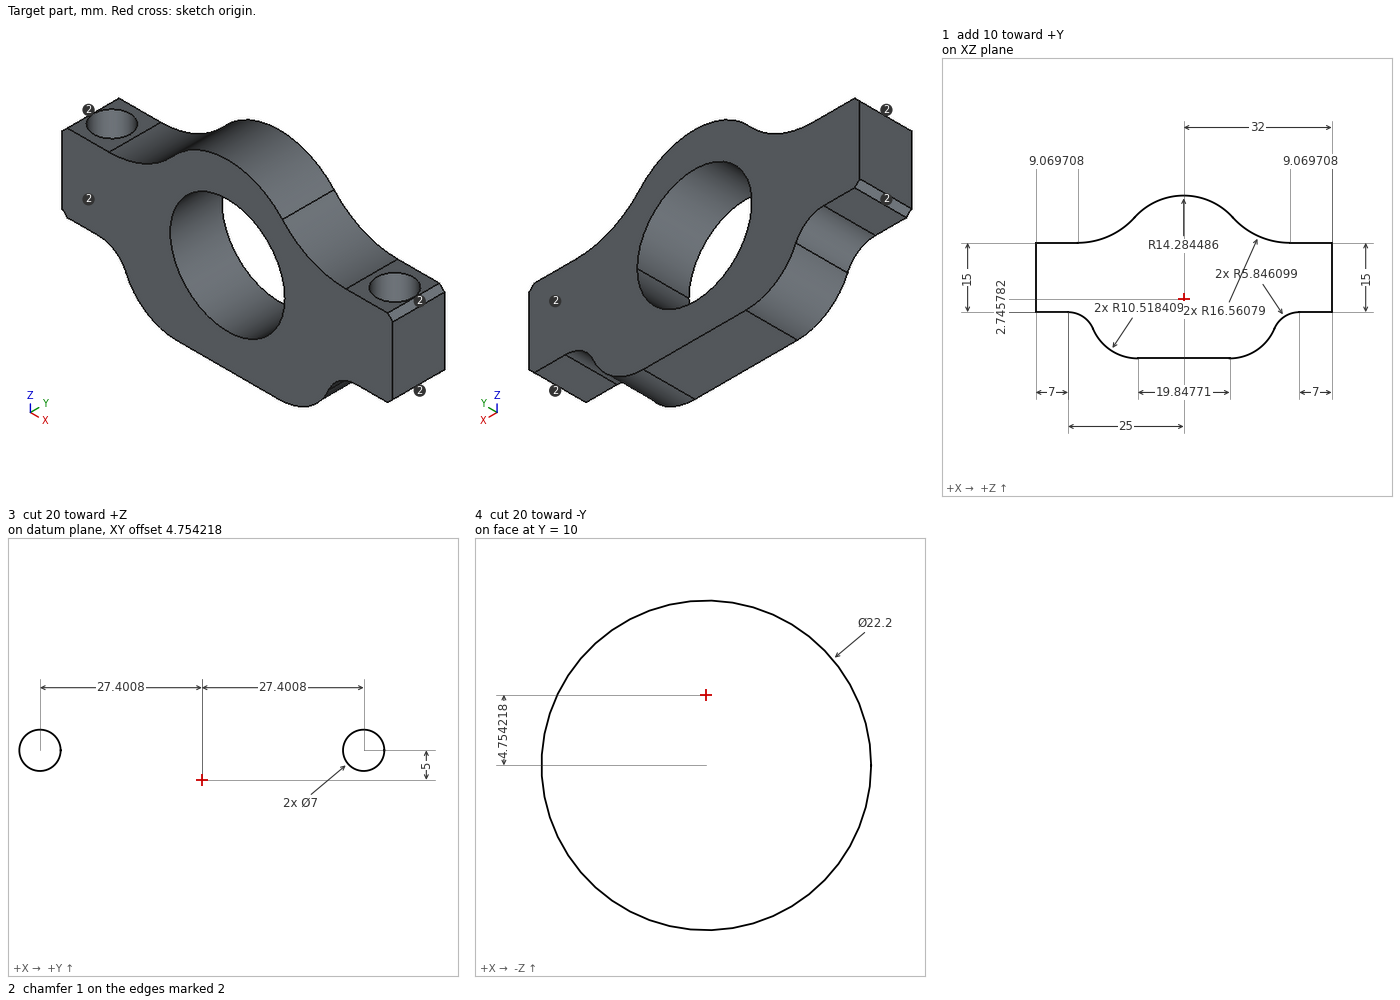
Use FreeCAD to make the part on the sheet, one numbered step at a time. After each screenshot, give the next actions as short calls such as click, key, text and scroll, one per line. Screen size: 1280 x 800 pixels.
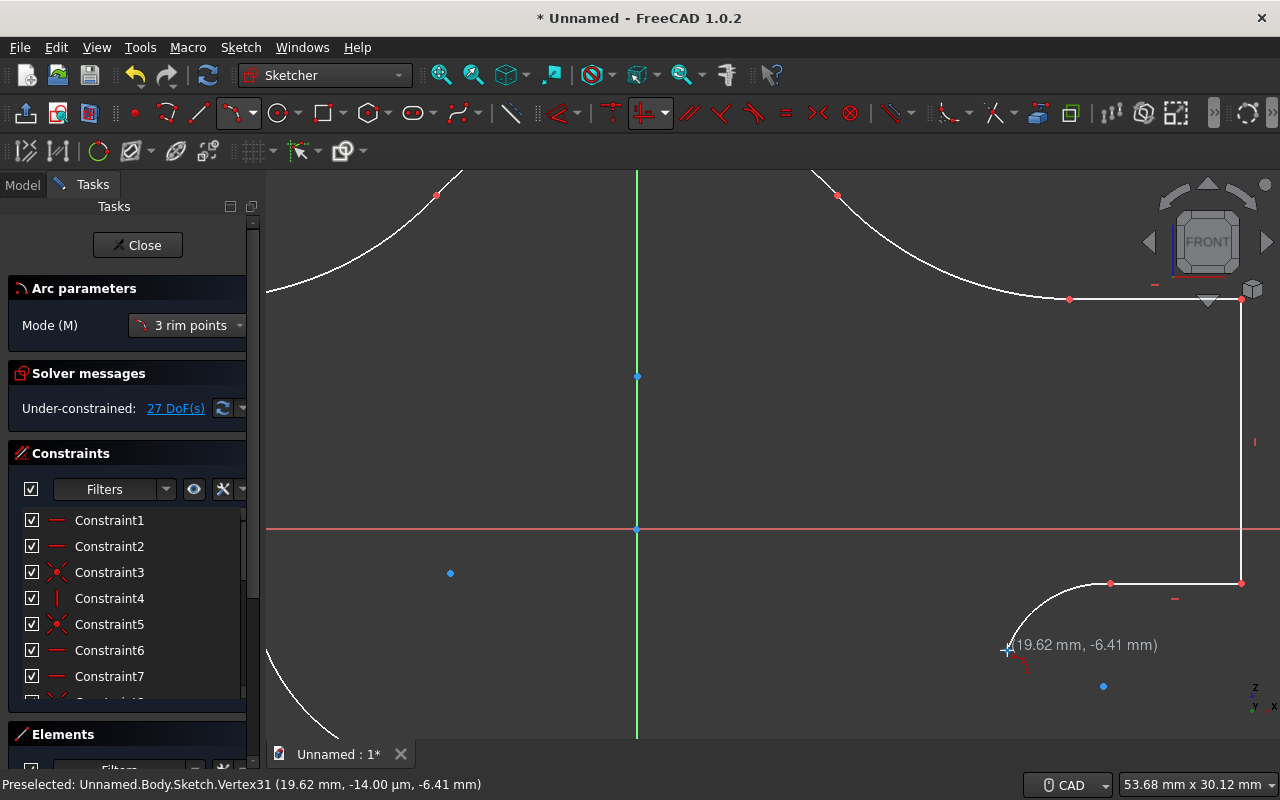
scroll(760, 468, down, 4)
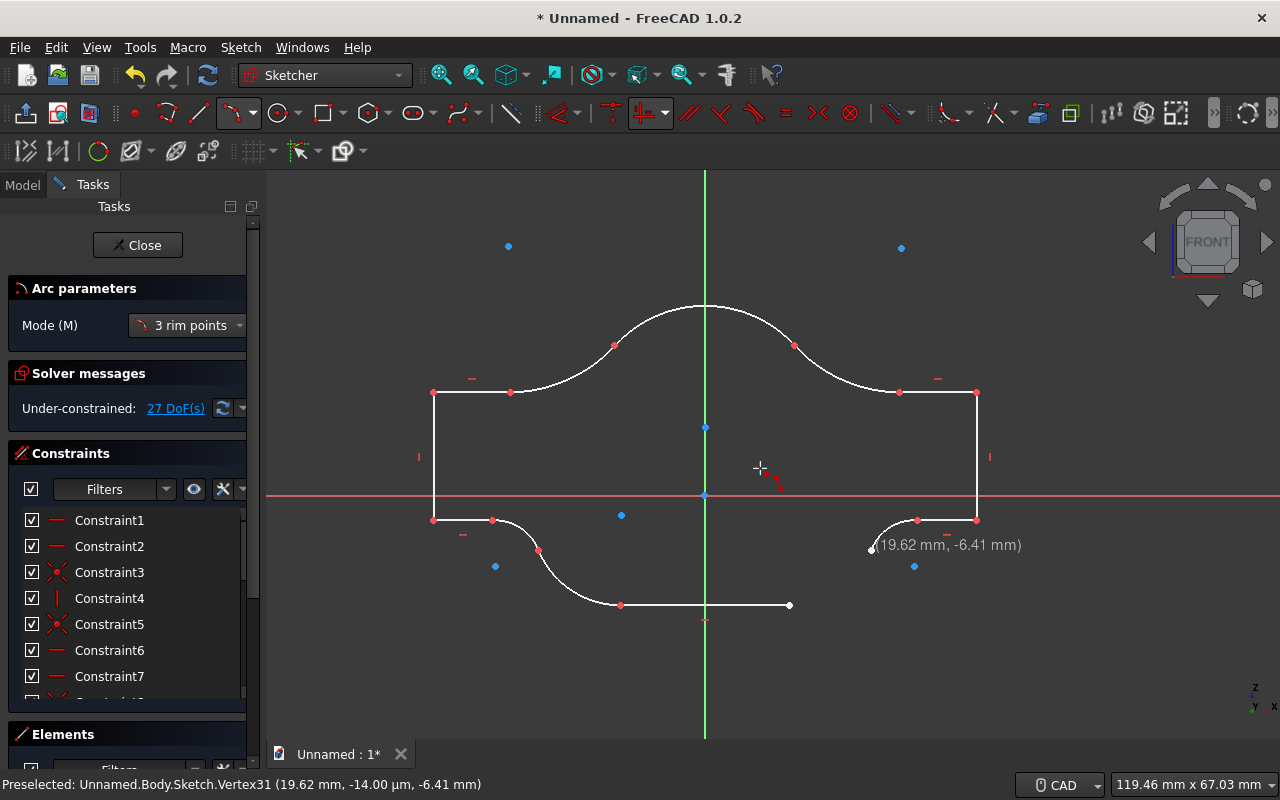
click(790, 605)
click(838, 589)
key(Escape)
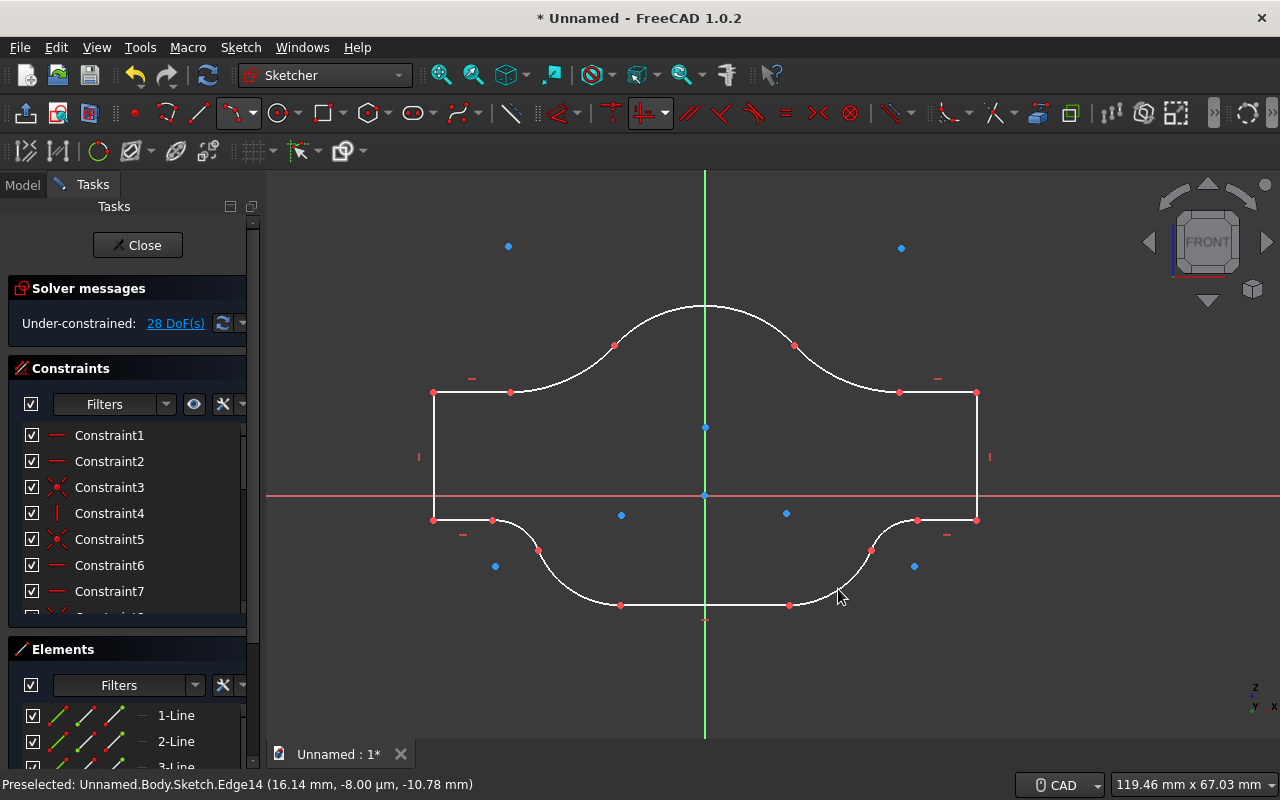
click(739, 605)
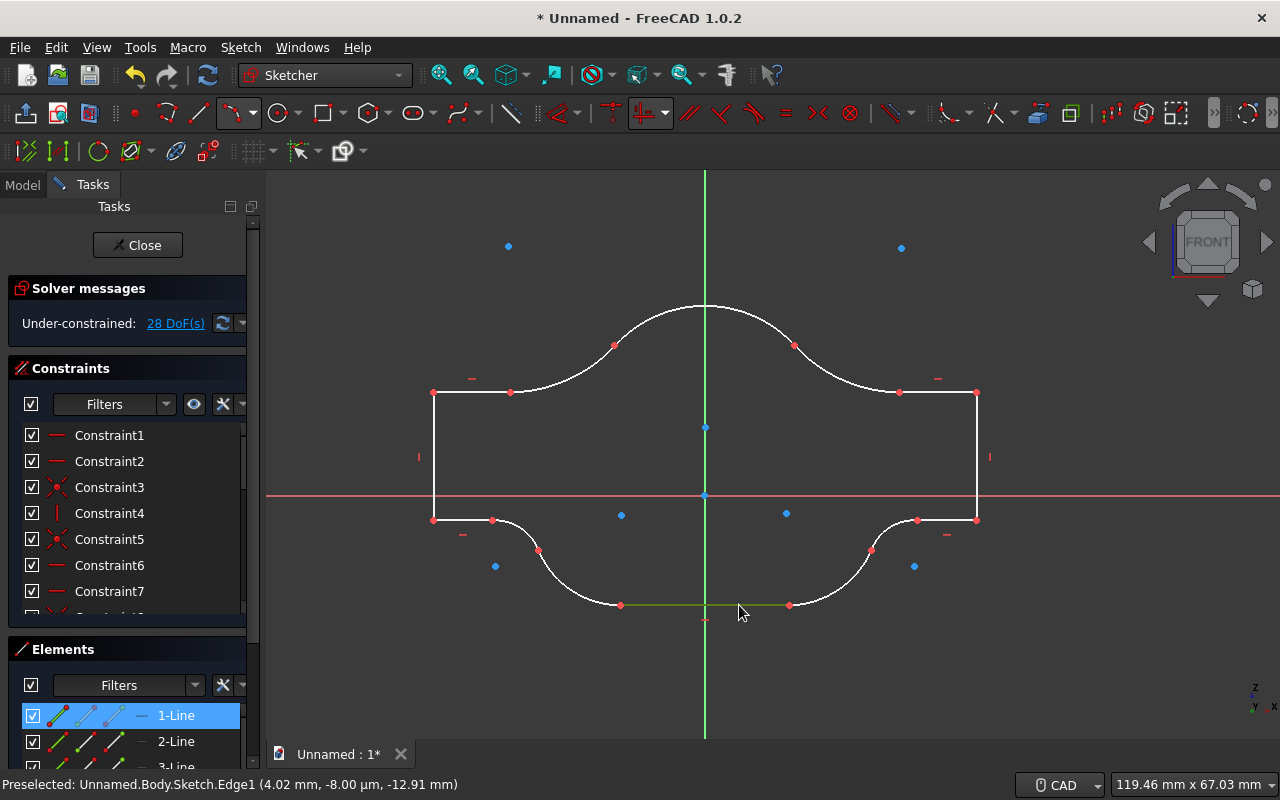
click(555, 577)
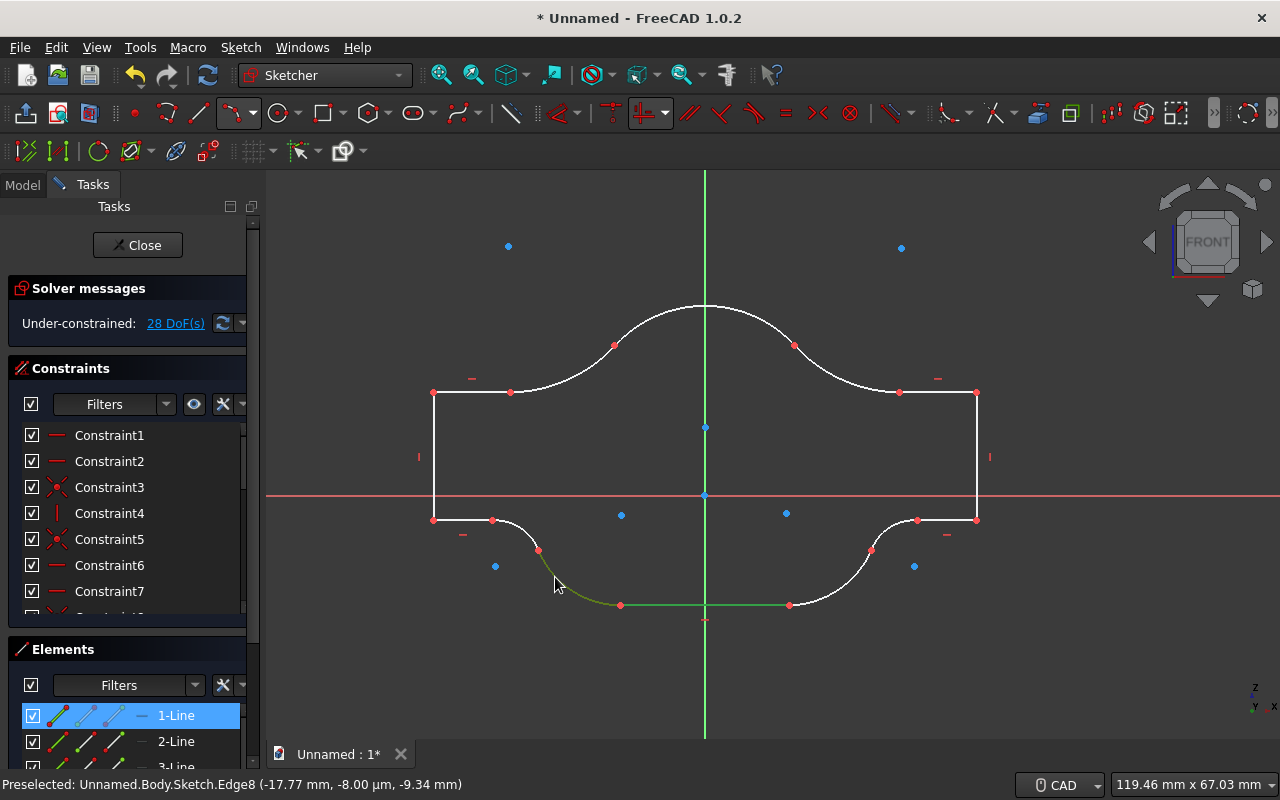
click(754, 114)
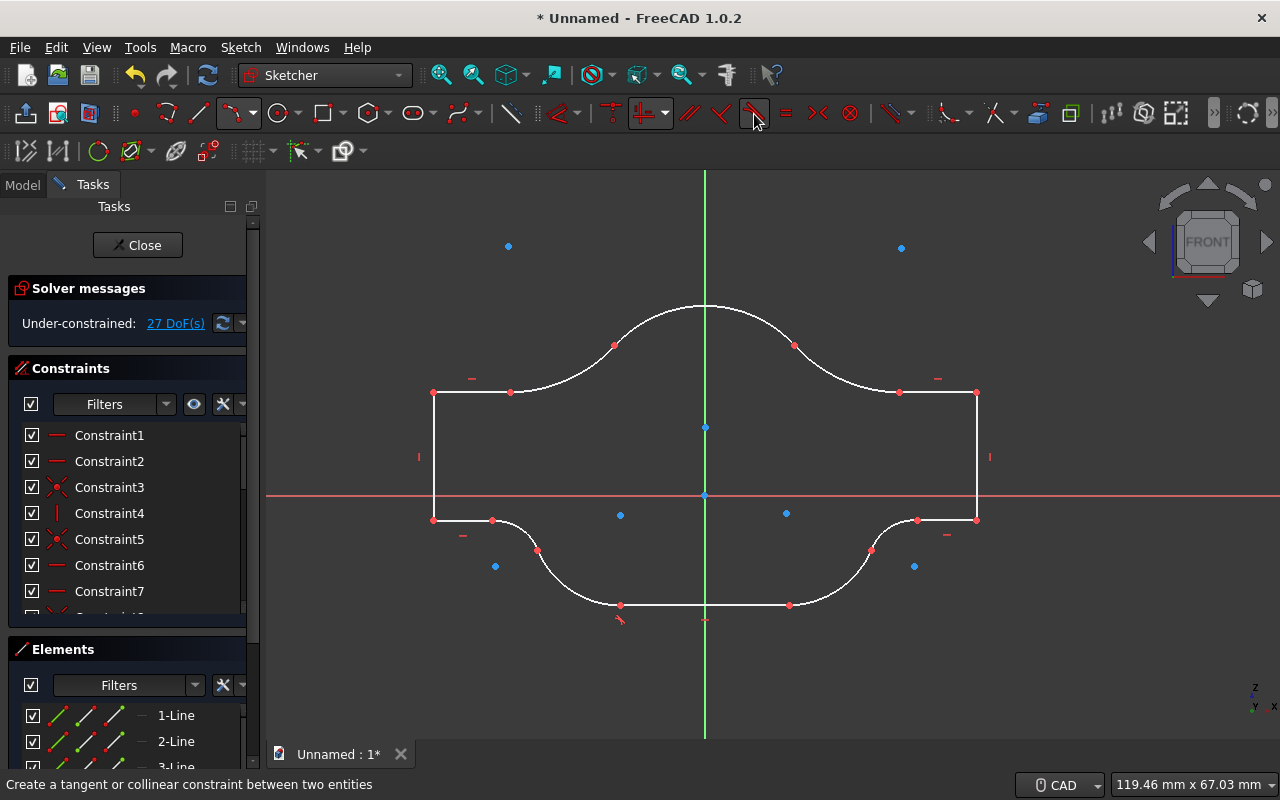
click(739, 605)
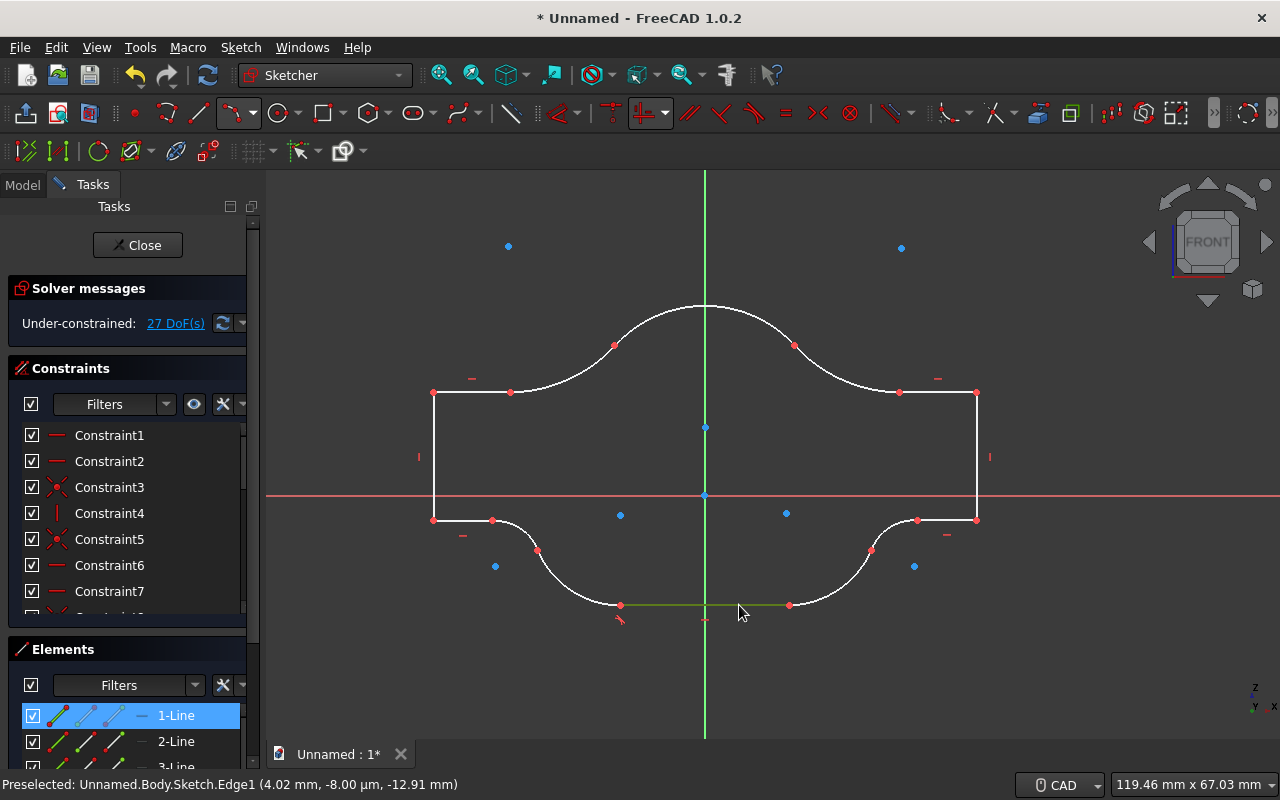
click(820, 599)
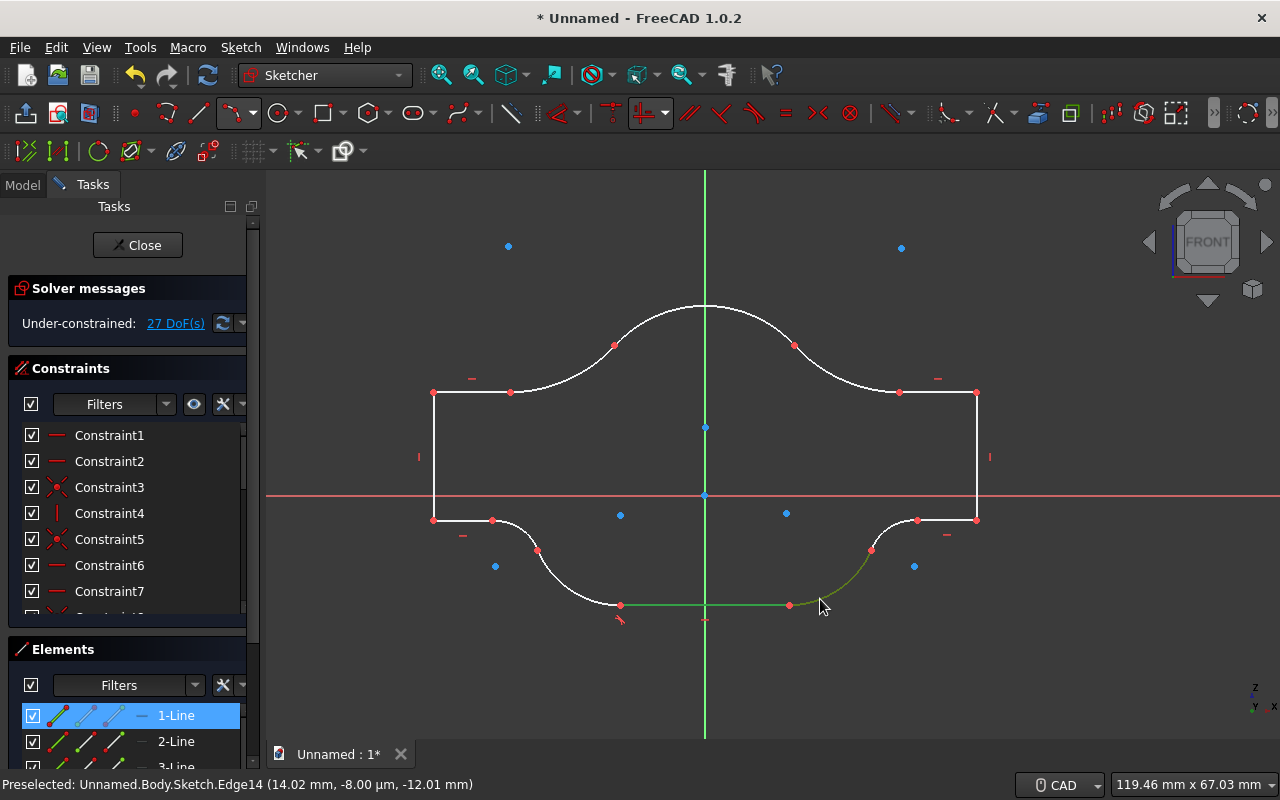
click(754, 114)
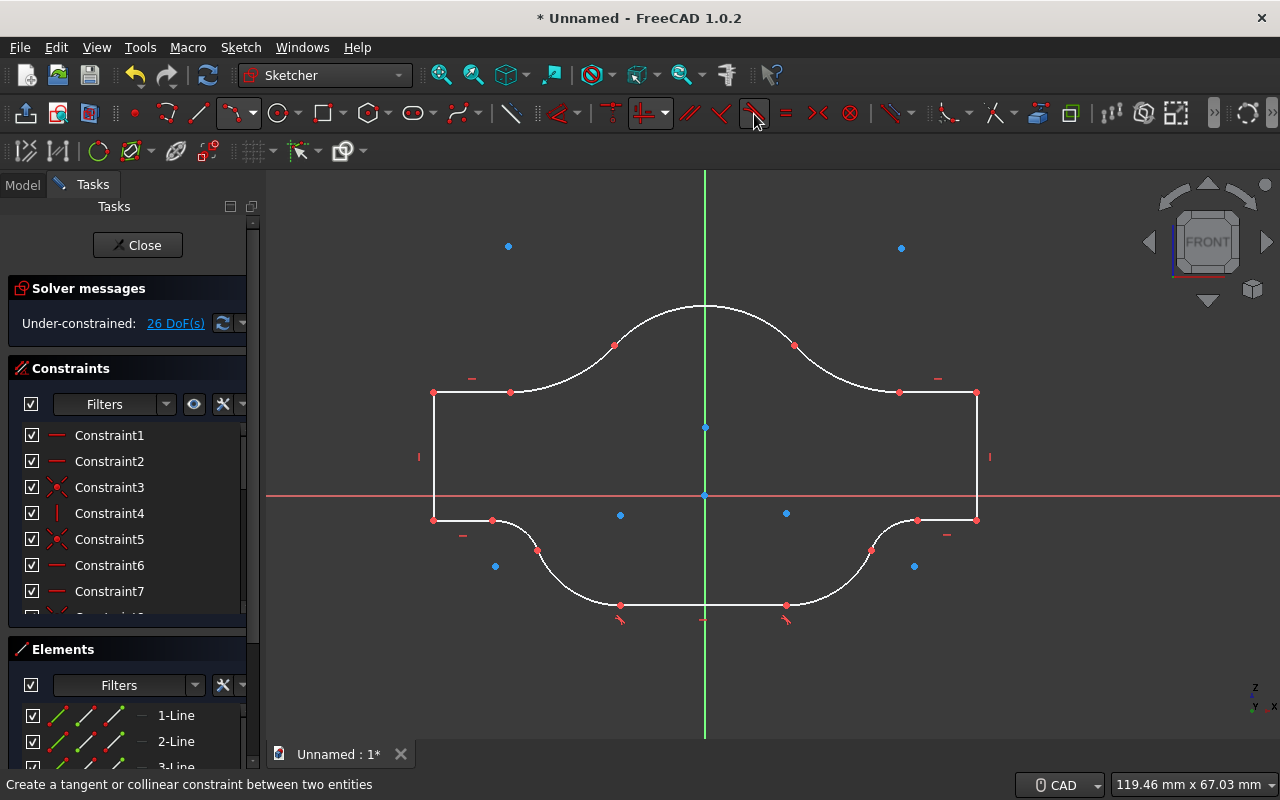
click(475, 521)